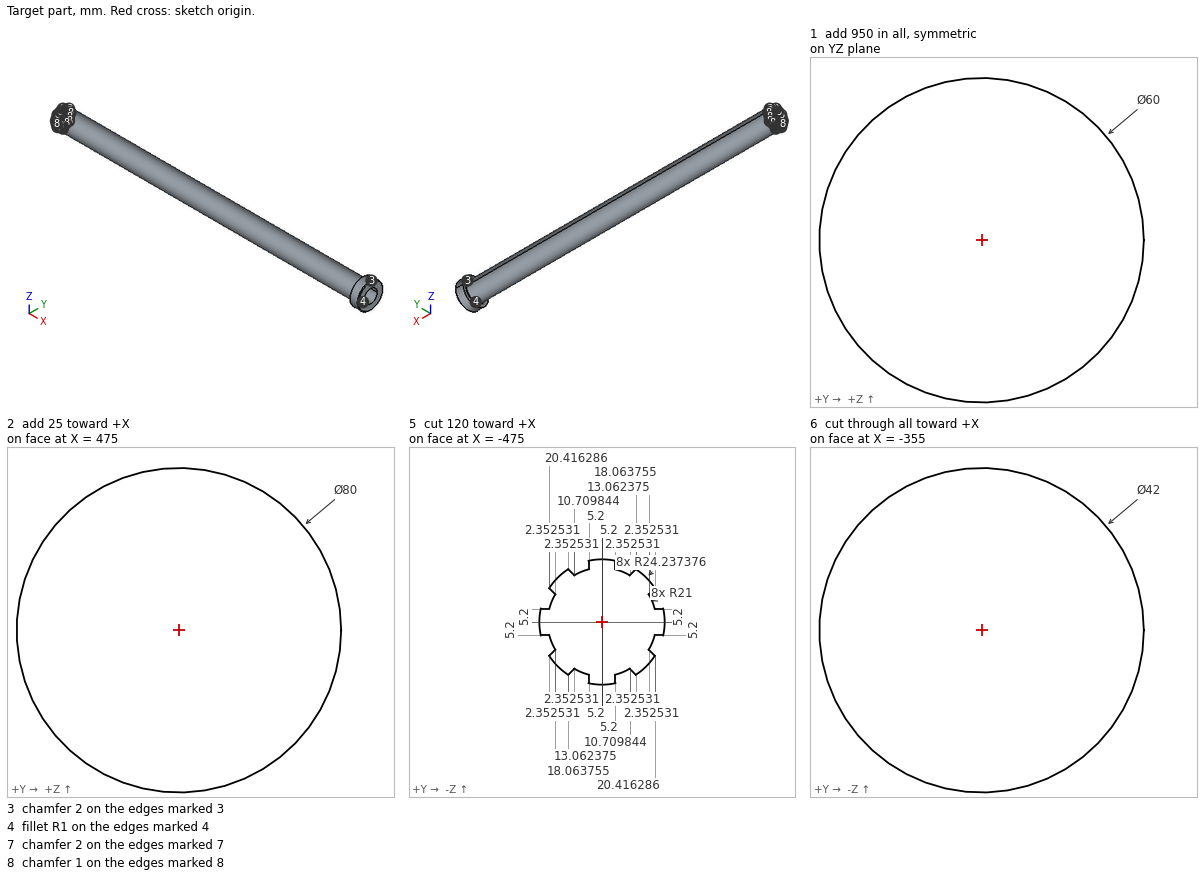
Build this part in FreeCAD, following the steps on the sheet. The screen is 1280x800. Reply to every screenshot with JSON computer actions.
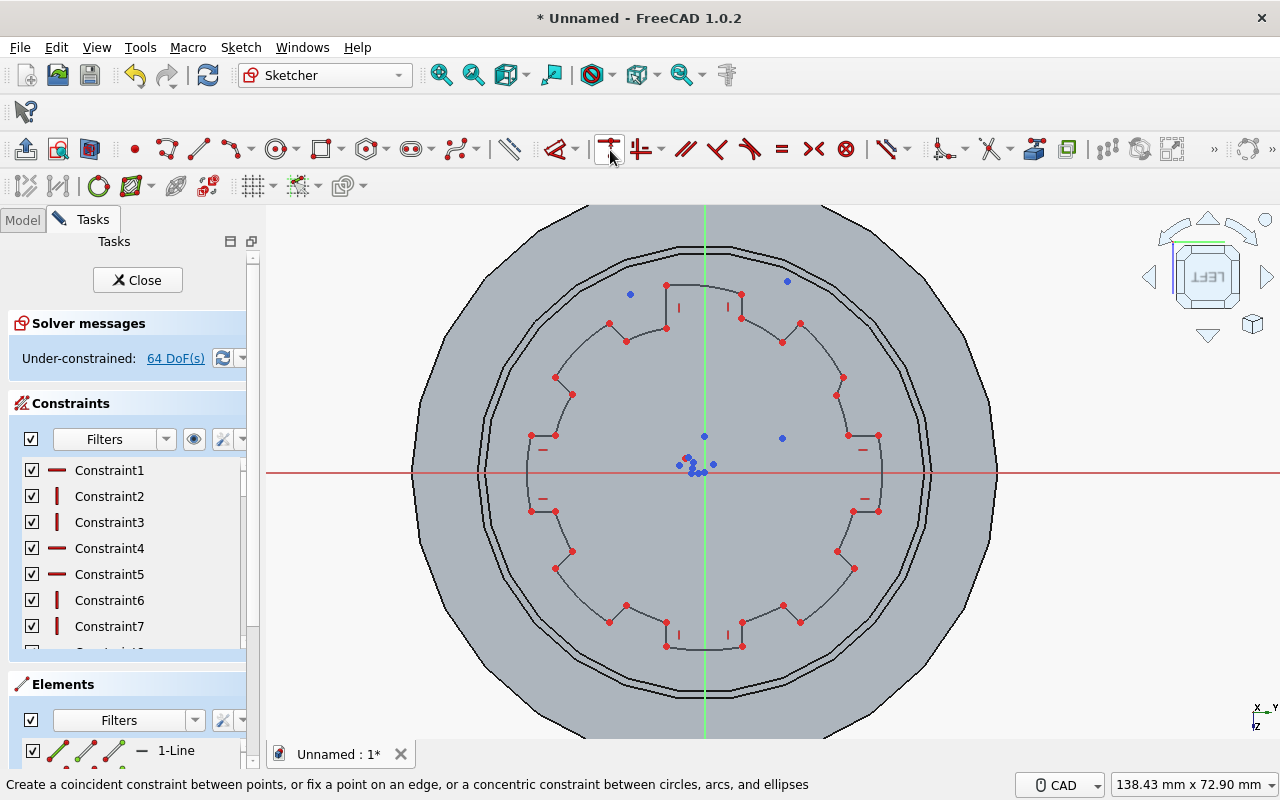
{"action": "left_click", "coordinate": [846, 423]}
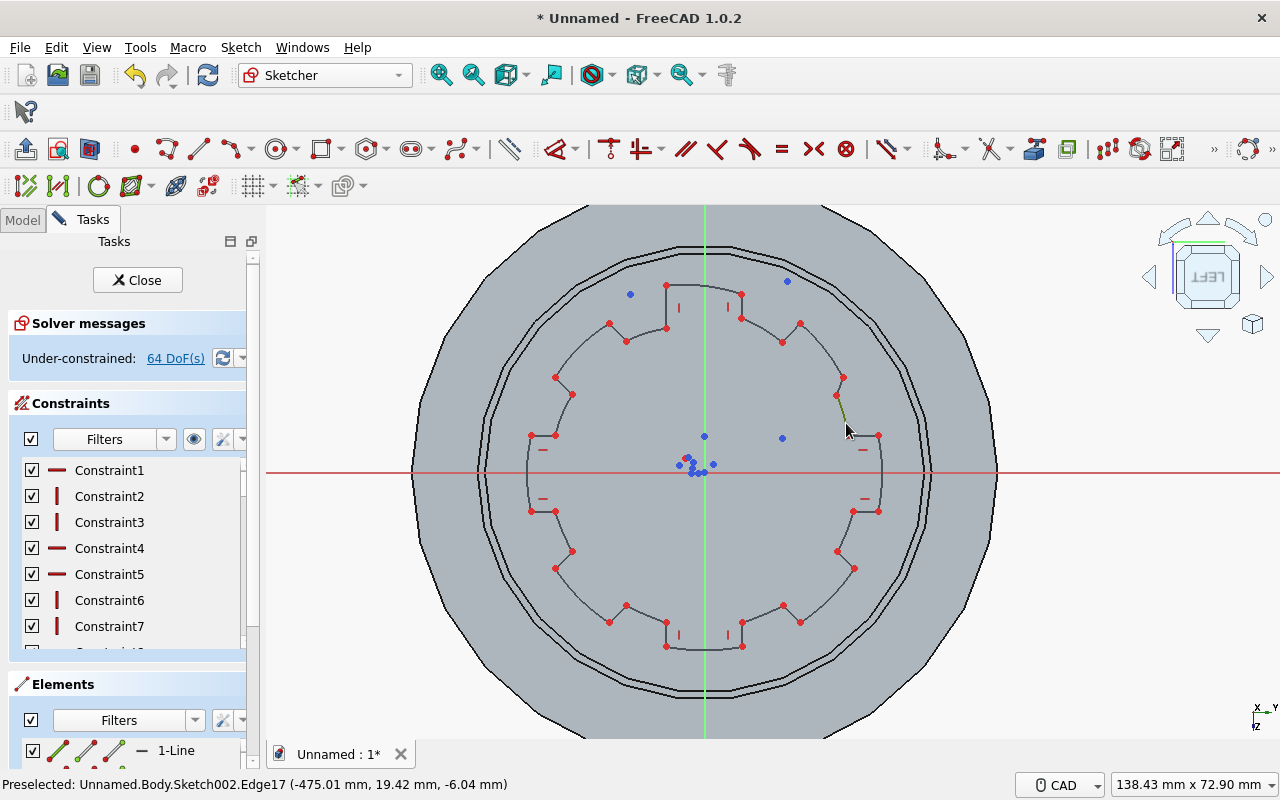
{"action": "left_click", "coordinate": [590, 337]}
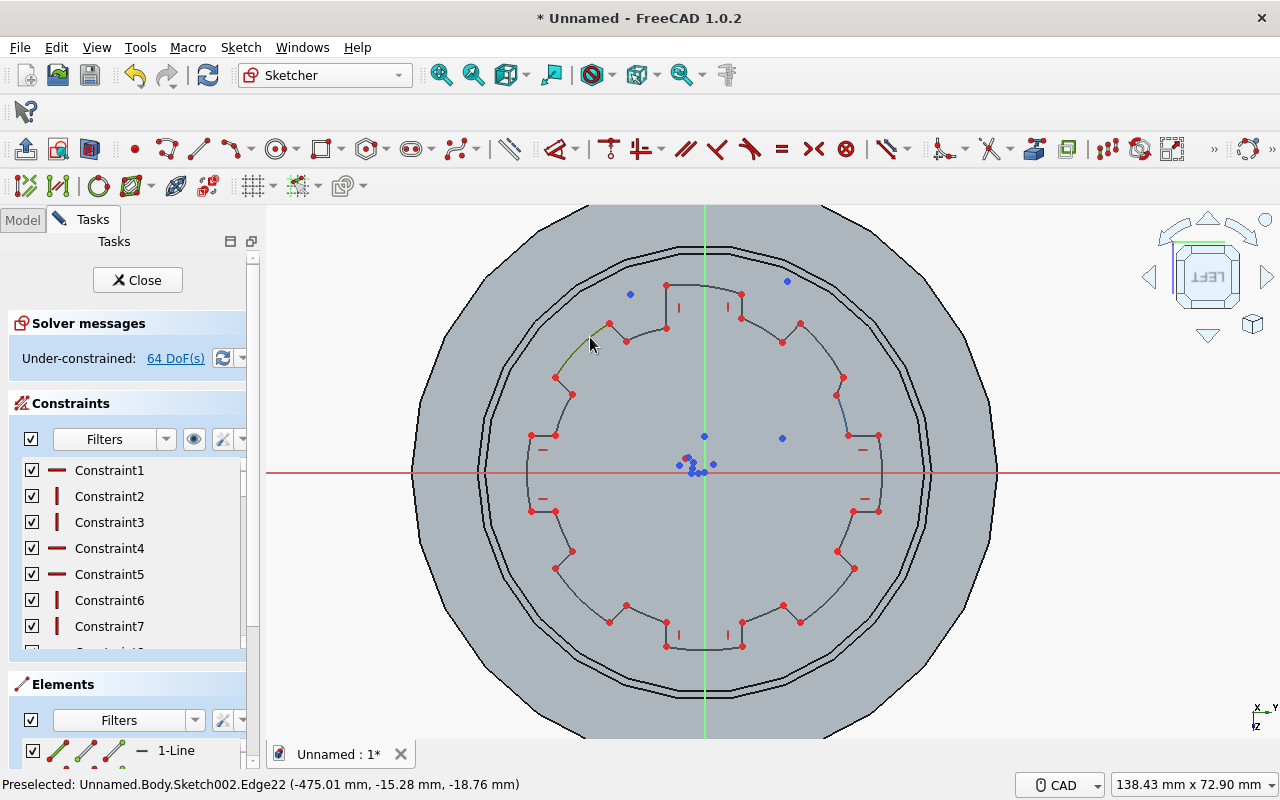
{"action": "left_click", "coordinate": [610, 150]}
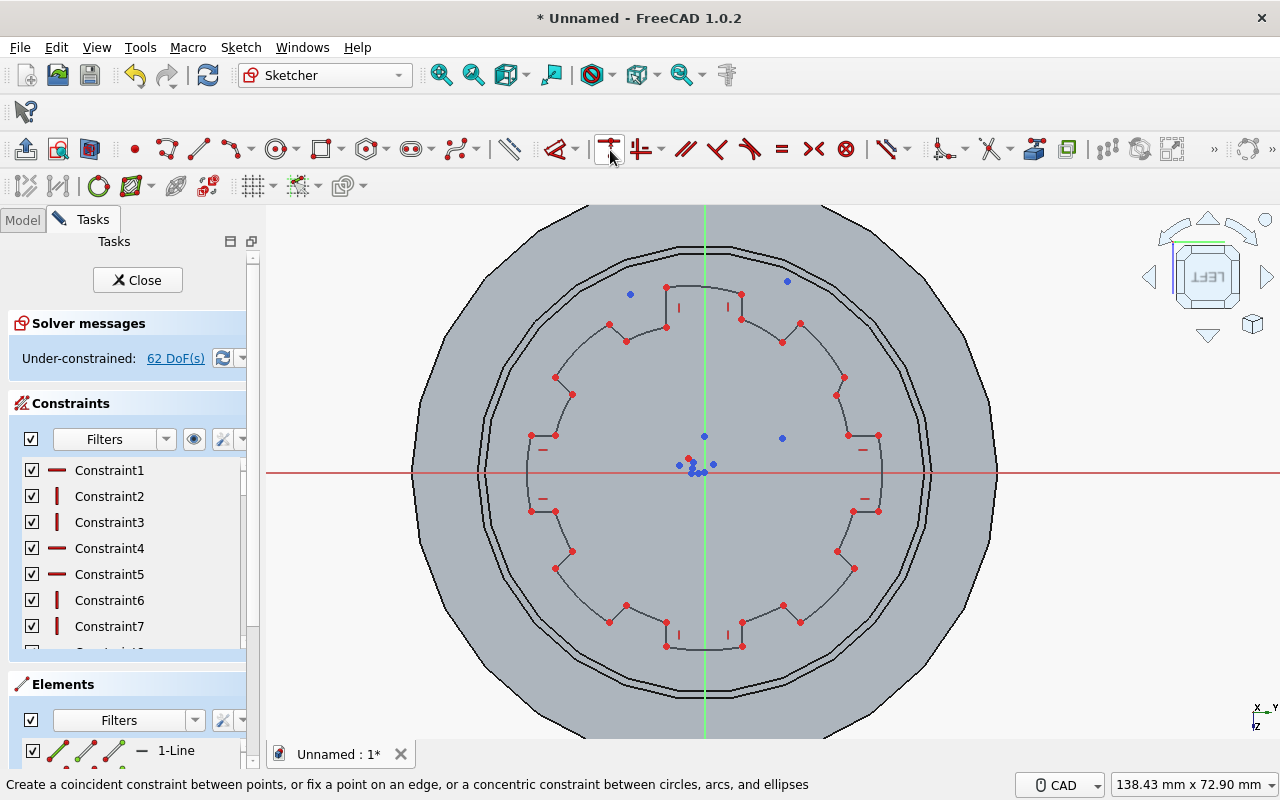
{"action": "left_click", "coordinate": [846, 423]}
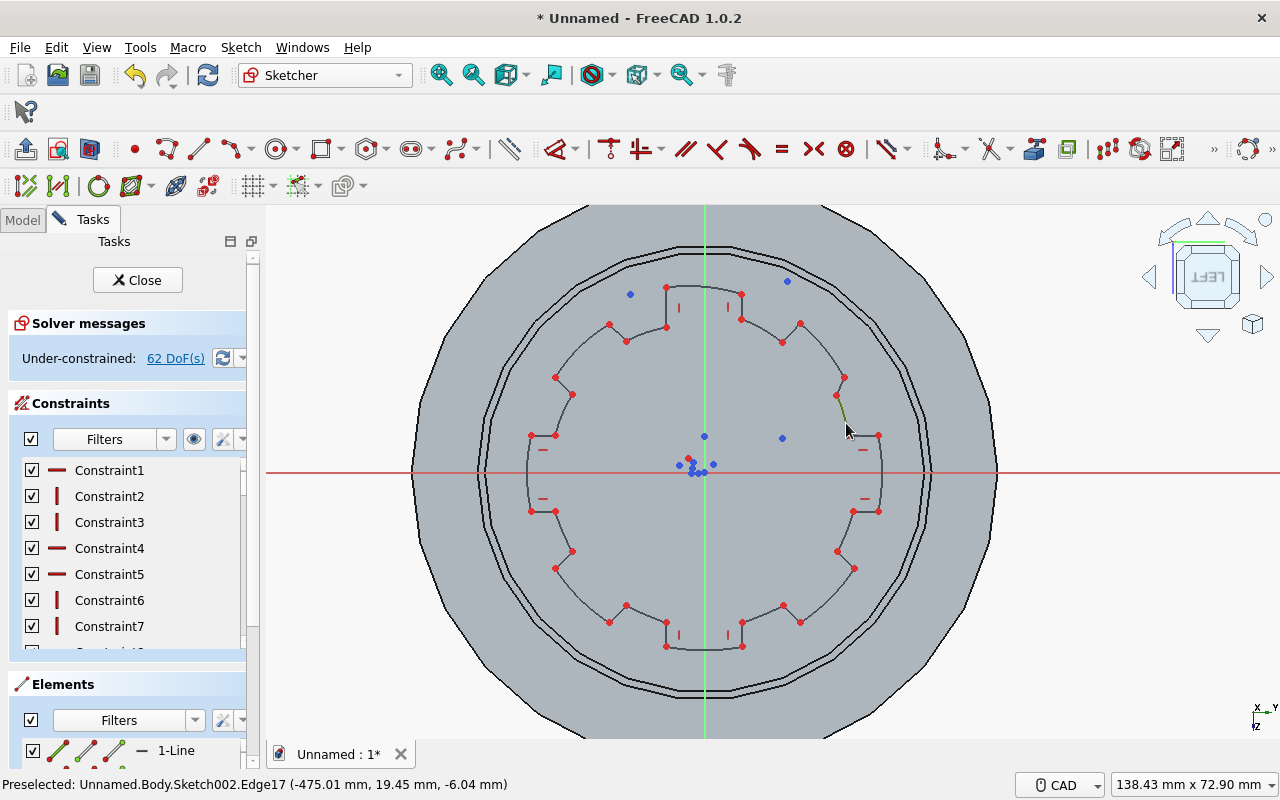
{"action": "left_click", "coordinate": [566, 407]}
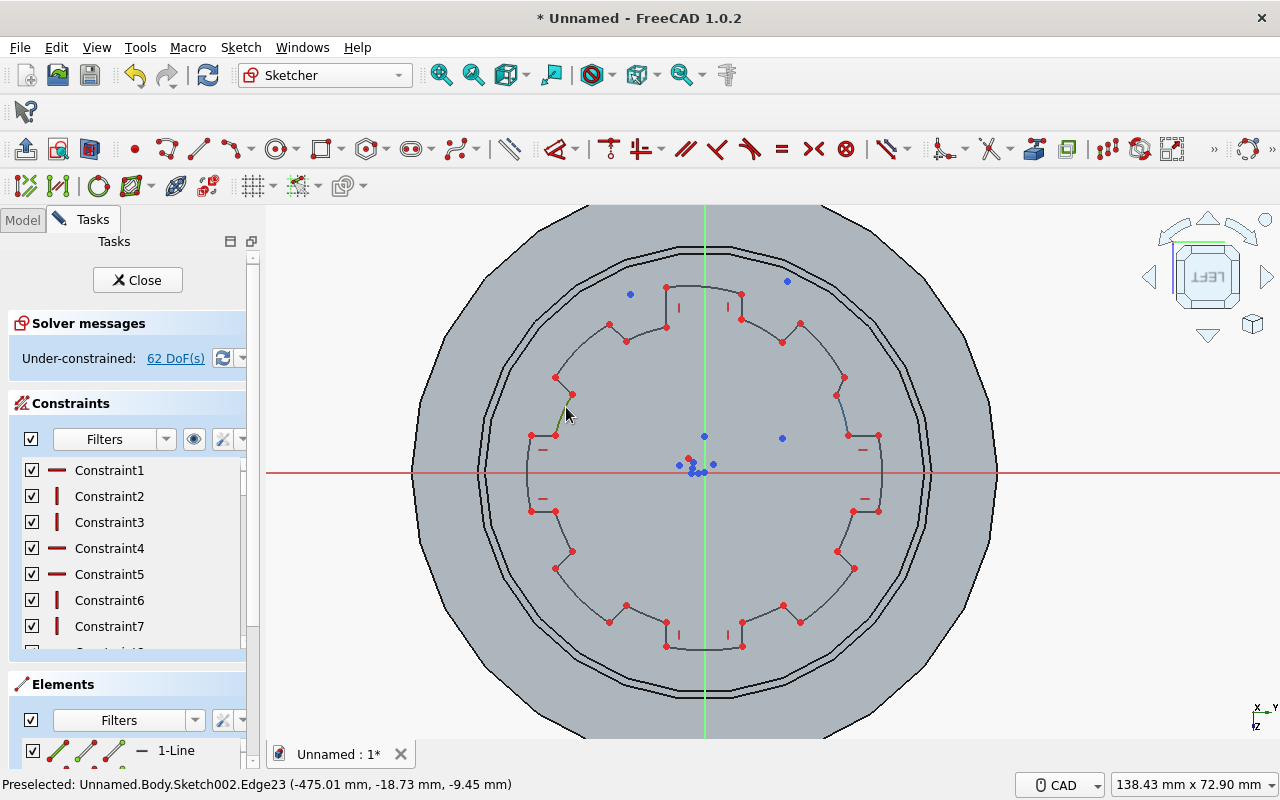
{"action": "left_click", "coordinate": [610, 150]}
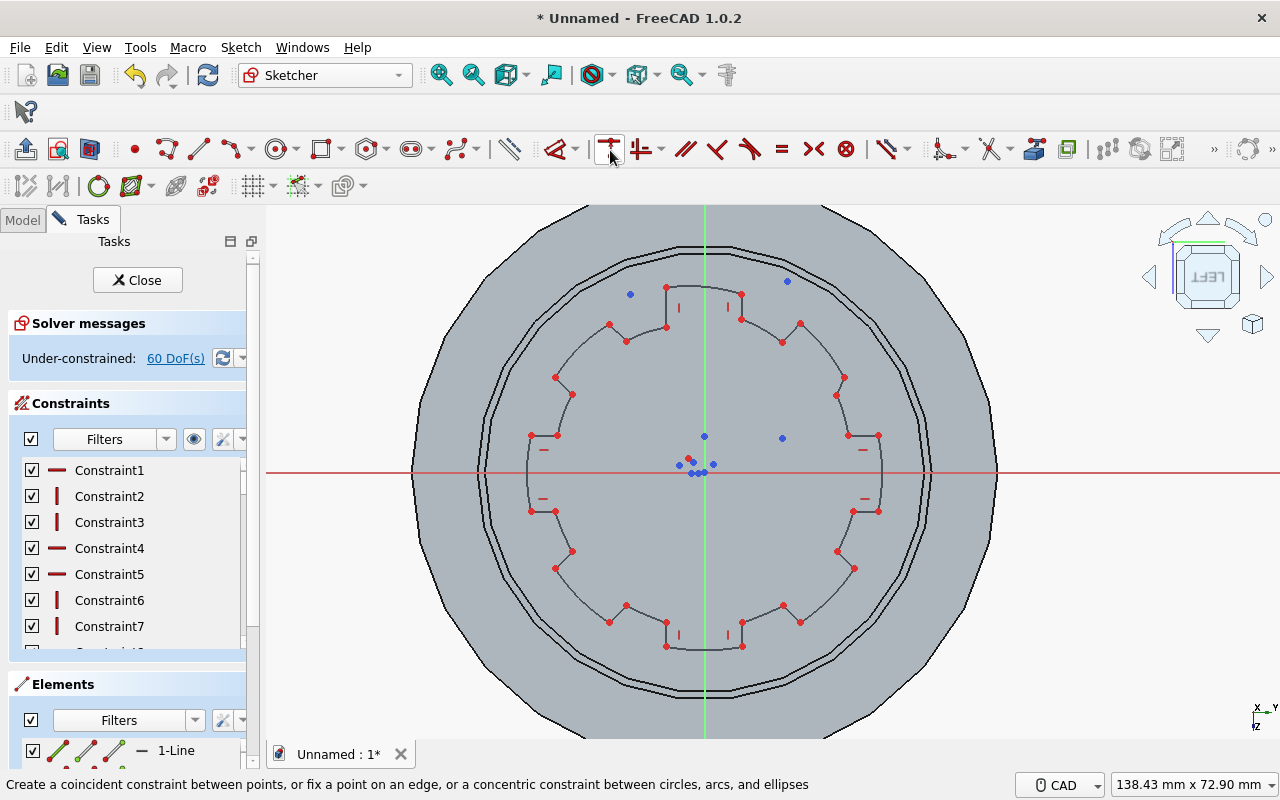
{"action": "left_click", "coordinate": [846, 423]}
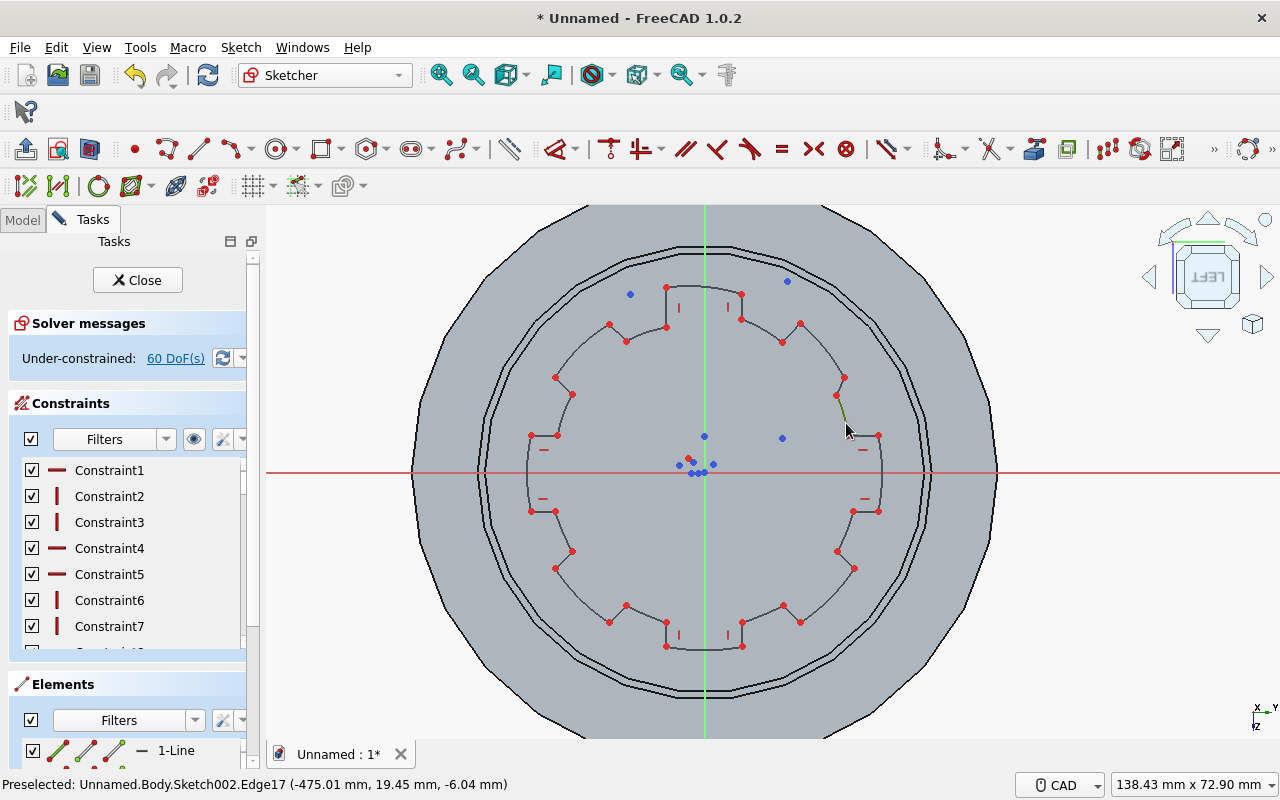
{"action": "left_click", "coordinate": [528, 459]}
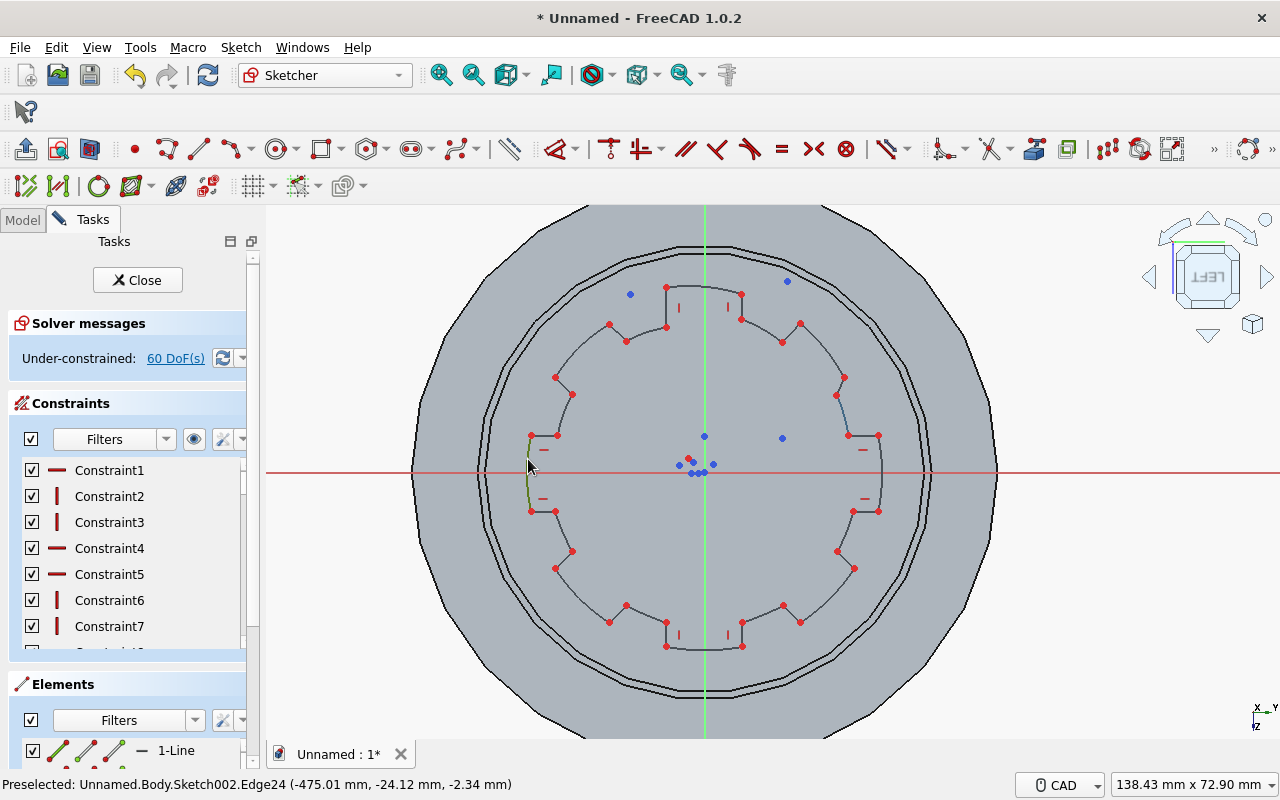
{"action": "key", "text": "c"}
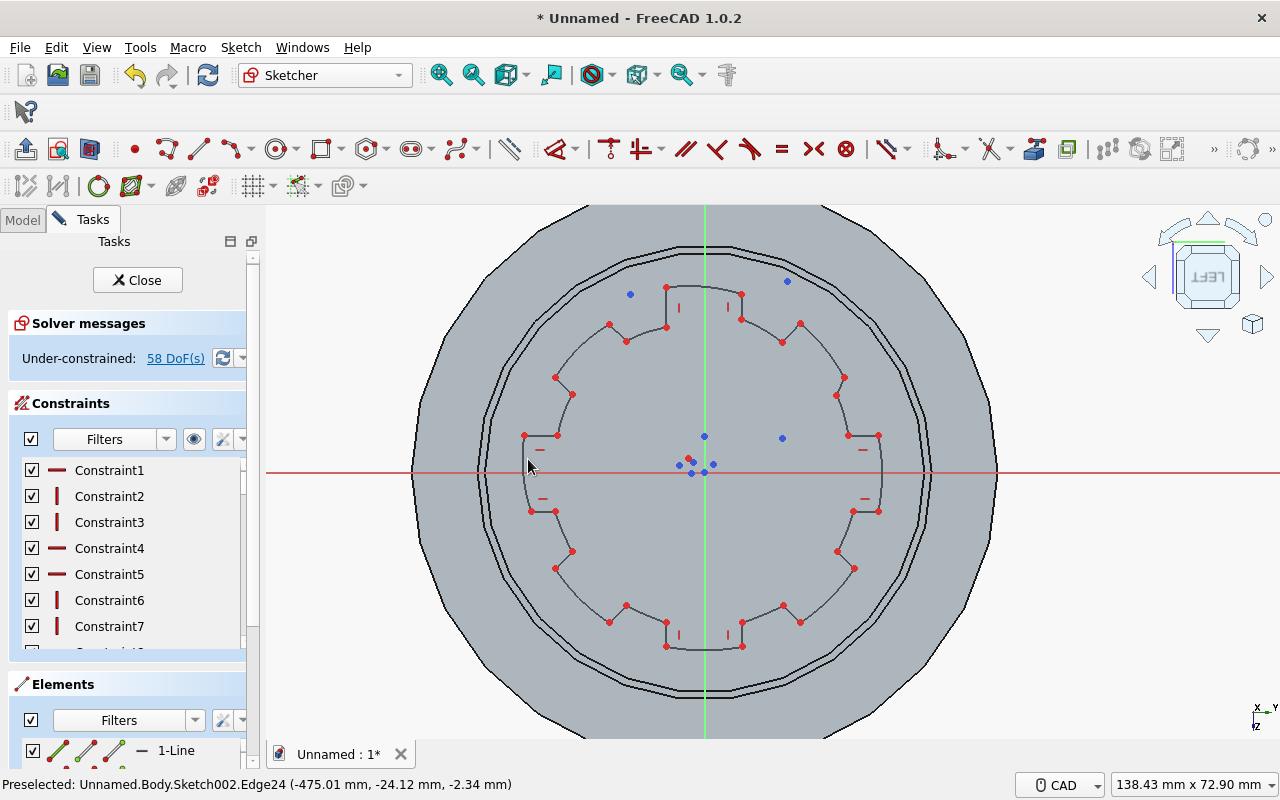
{"action": "left_click", "coordinate": [846, 423]}